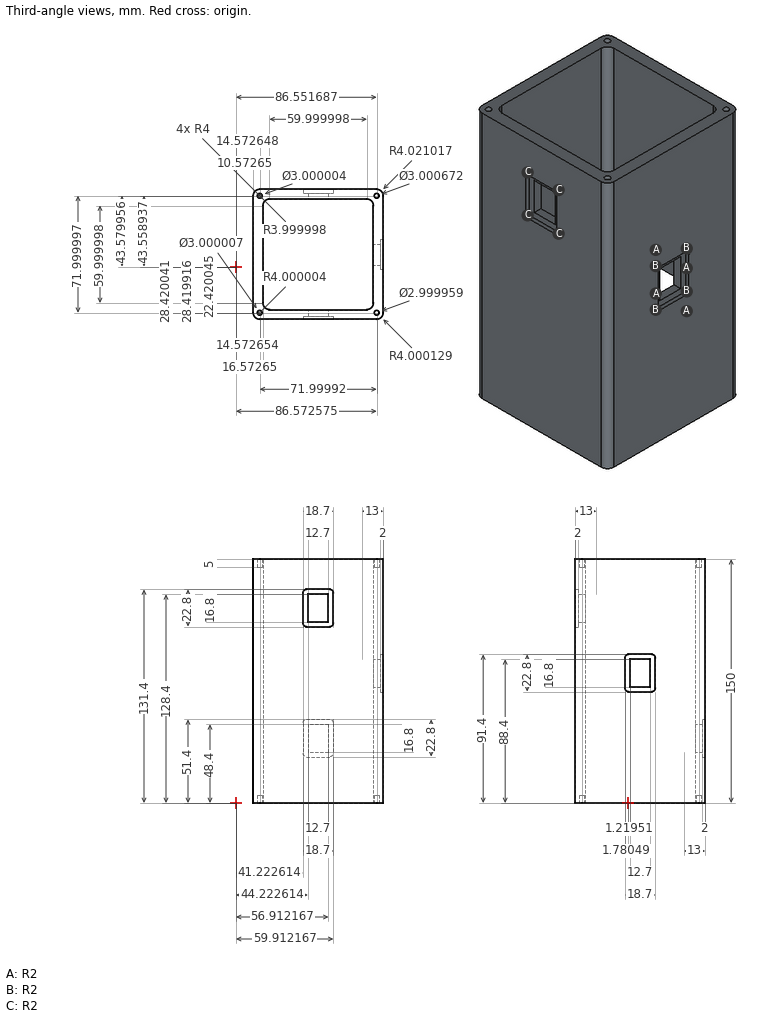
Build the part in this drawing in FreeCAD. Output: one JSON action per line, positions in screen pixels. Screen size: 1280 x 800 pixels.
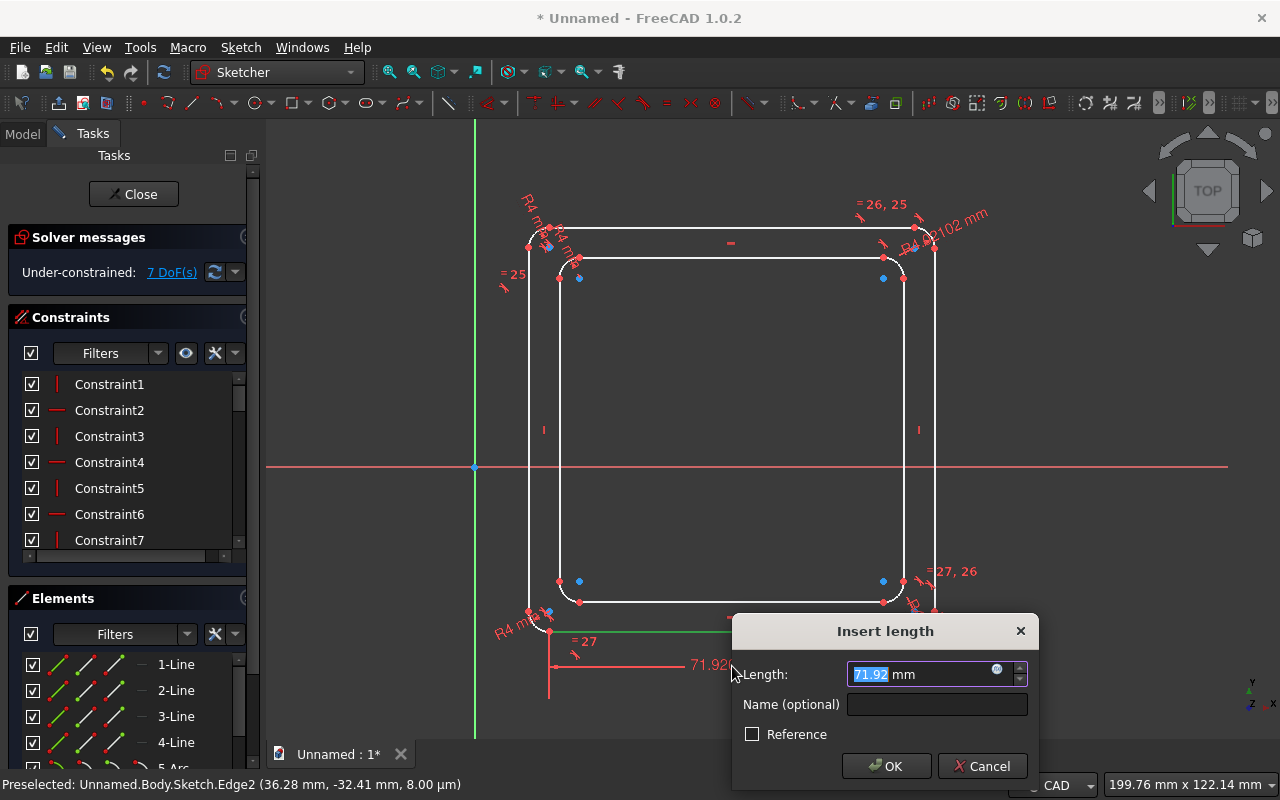
{"action": "type", "text": "71.99992"}
{"action": "key", "text": "Return"}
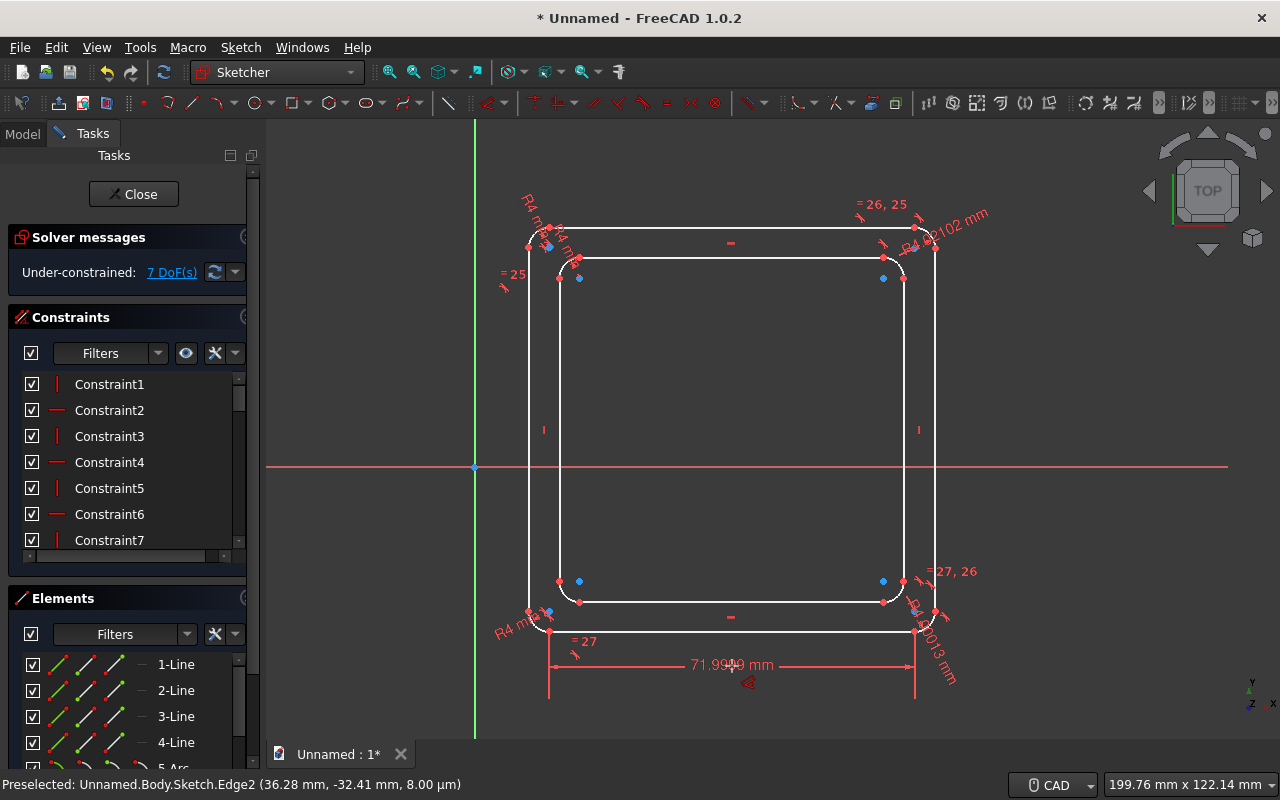
{"action": "left_click", "coordinate": [529, 357]}
{"action": "left_click", "coordinate": [495, 430]}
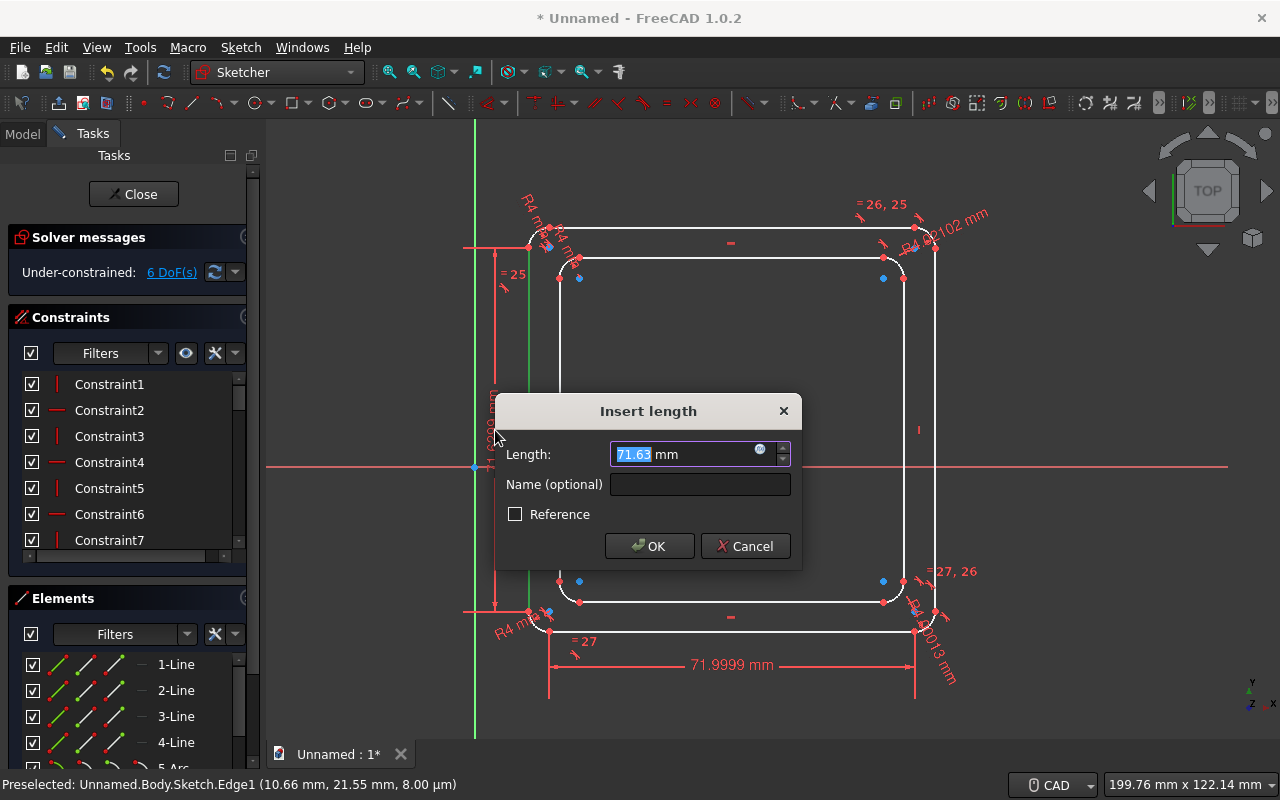
{"action": "type", "text": "71.999997"}
{"action": "key", "text": "Return"}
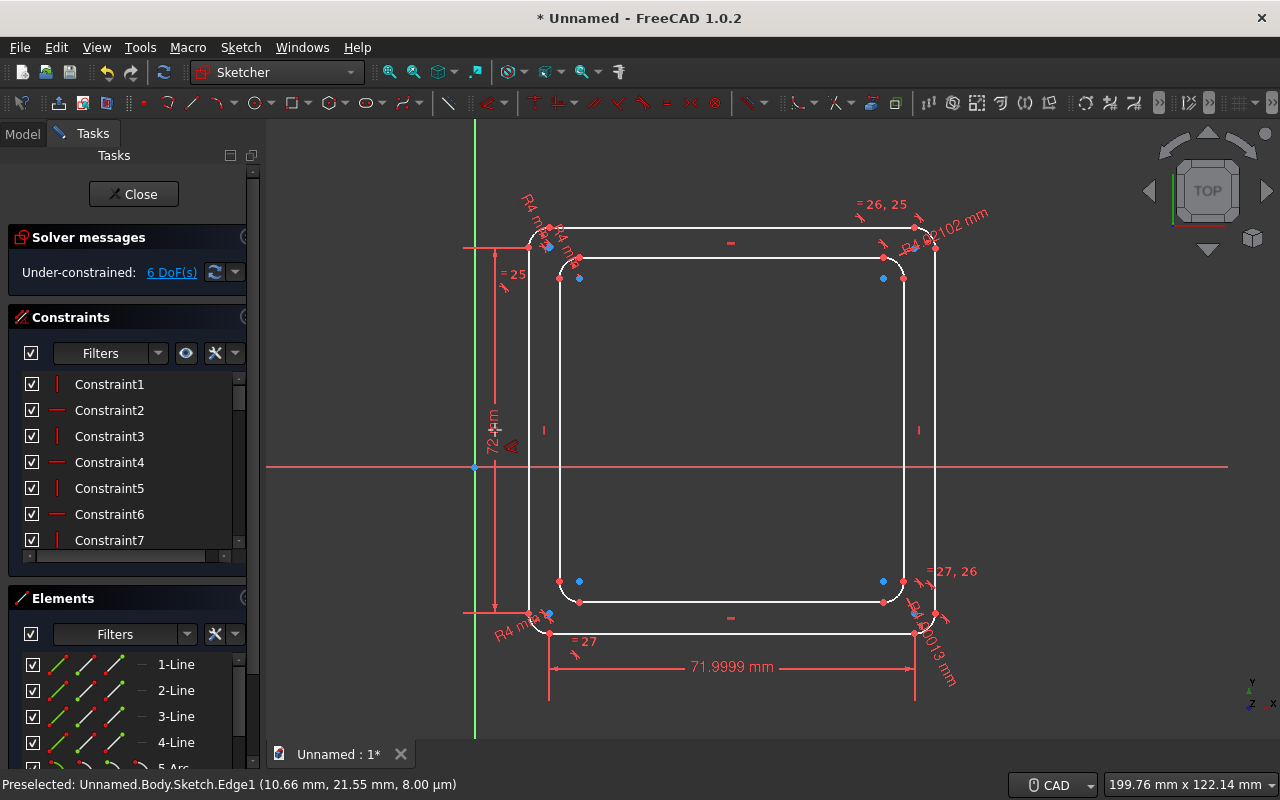
{"action": "left_click", "coordinate": [560, 491]}
{"action": "left_click", "coordinate": [594, 430]}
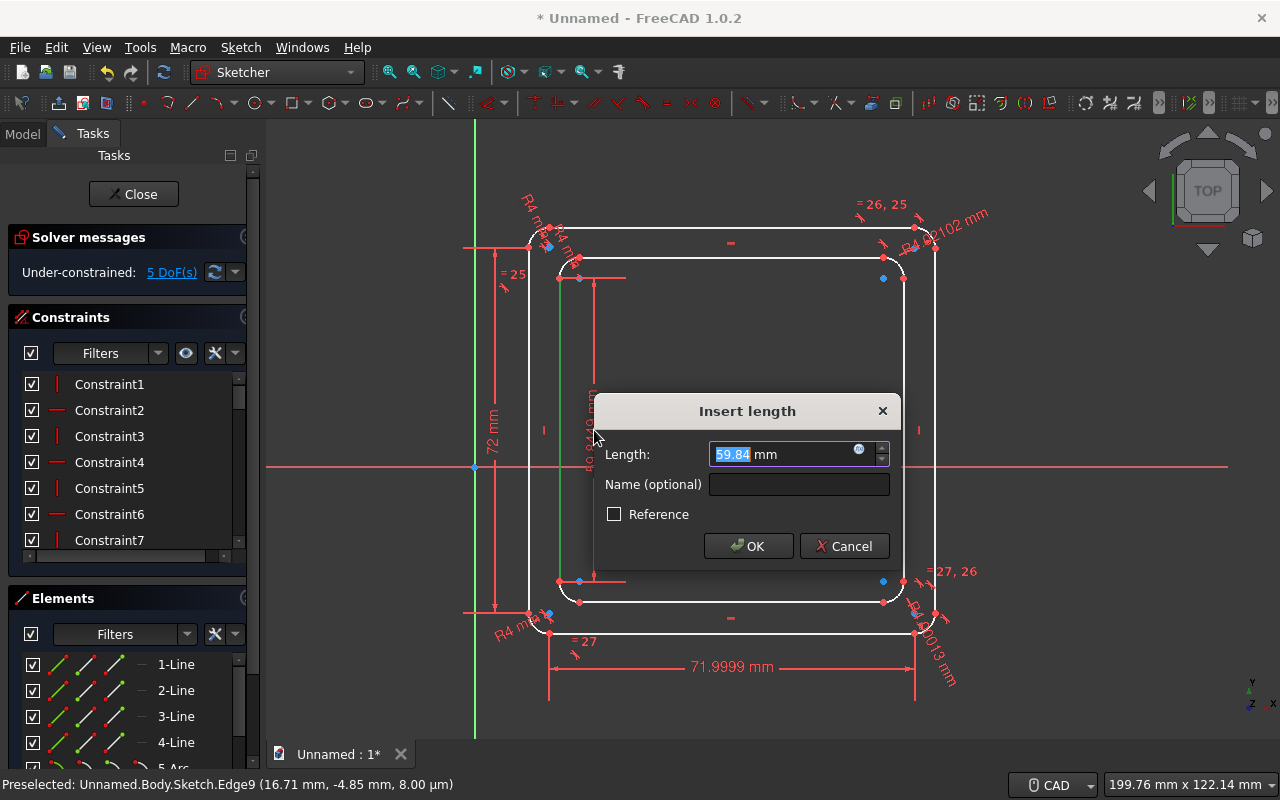
{"action": "type", "text": "59.999998"}
{"action": "key", "text": "Return"}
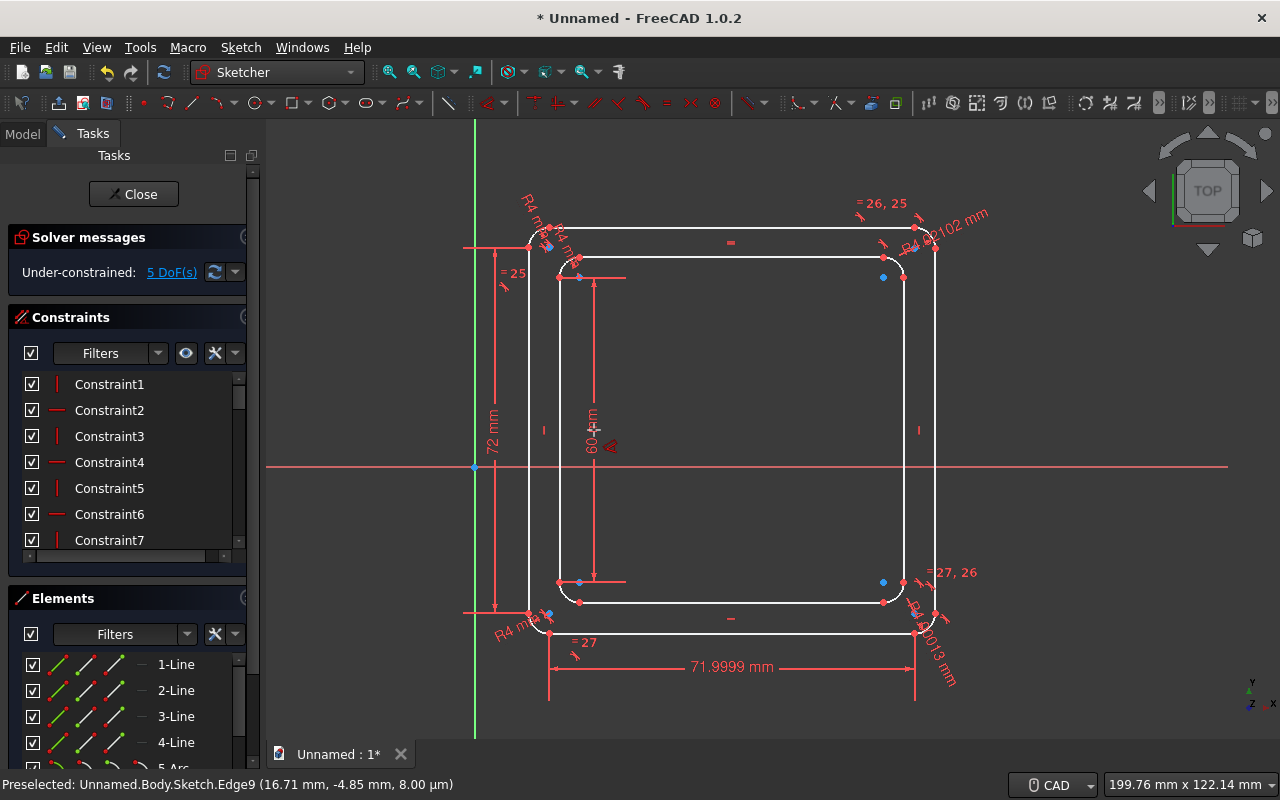
{"action": "left_click", "coordinate": [671, 257]}
{"action": "left_click", "coordinate": [732, 291]}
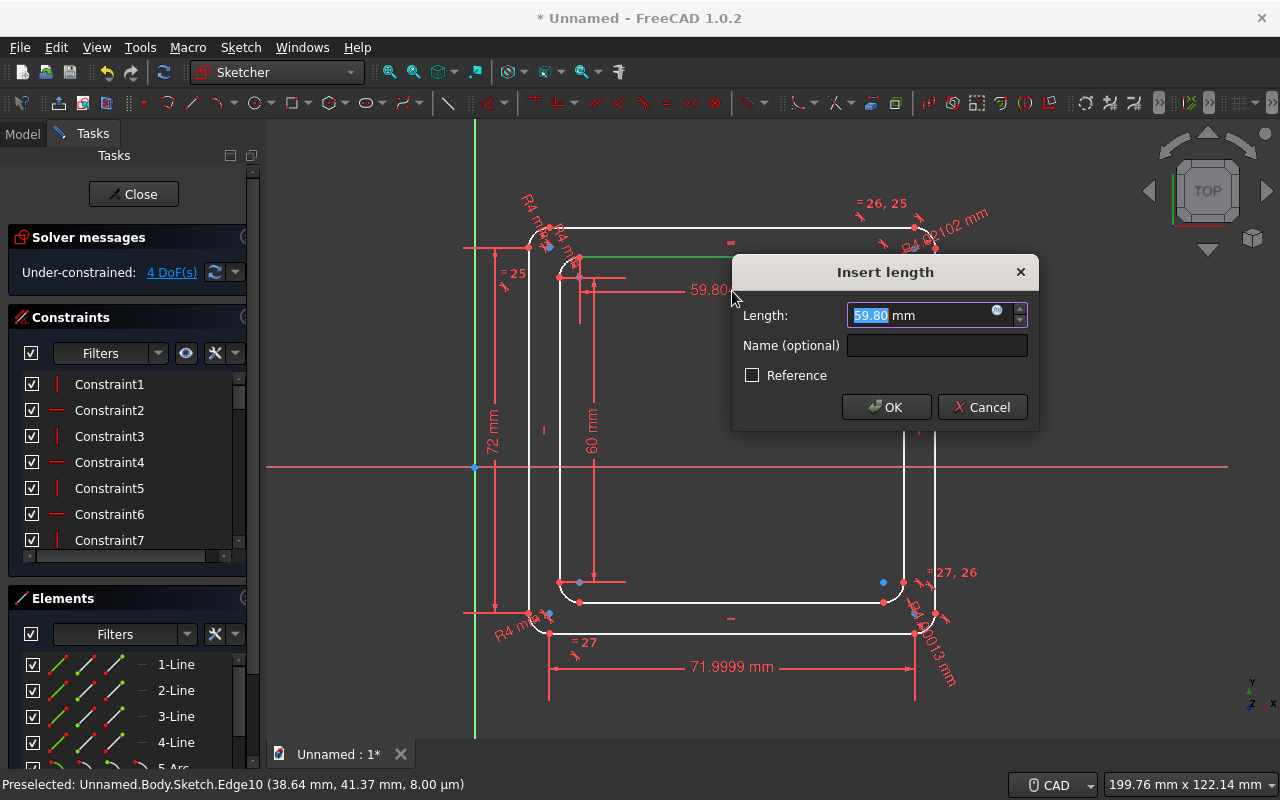
{"action": "type", "text": "59.999998"}
{"action": "key", "text": "Return"}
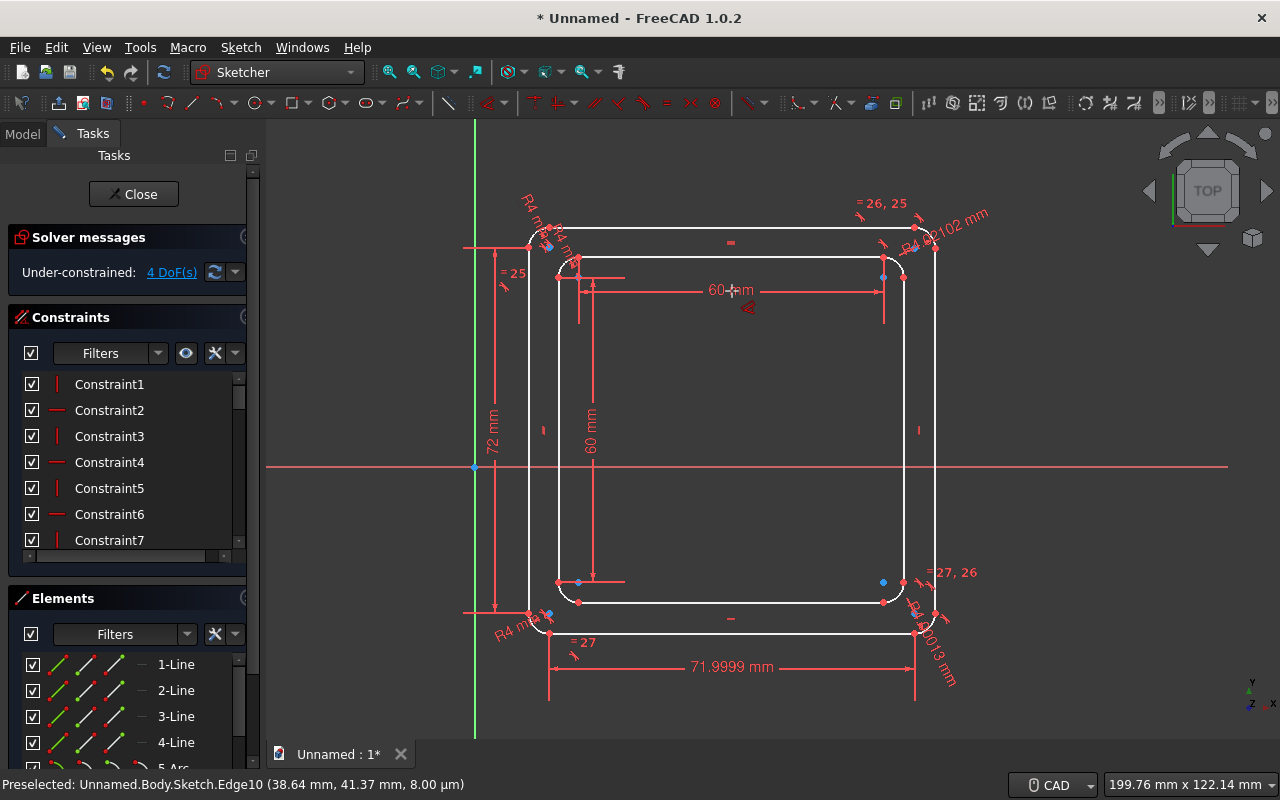
{"action": "left_click", "coordinate": [529, 248]}
{"action": "left_click", "coordinate": [502, 501]}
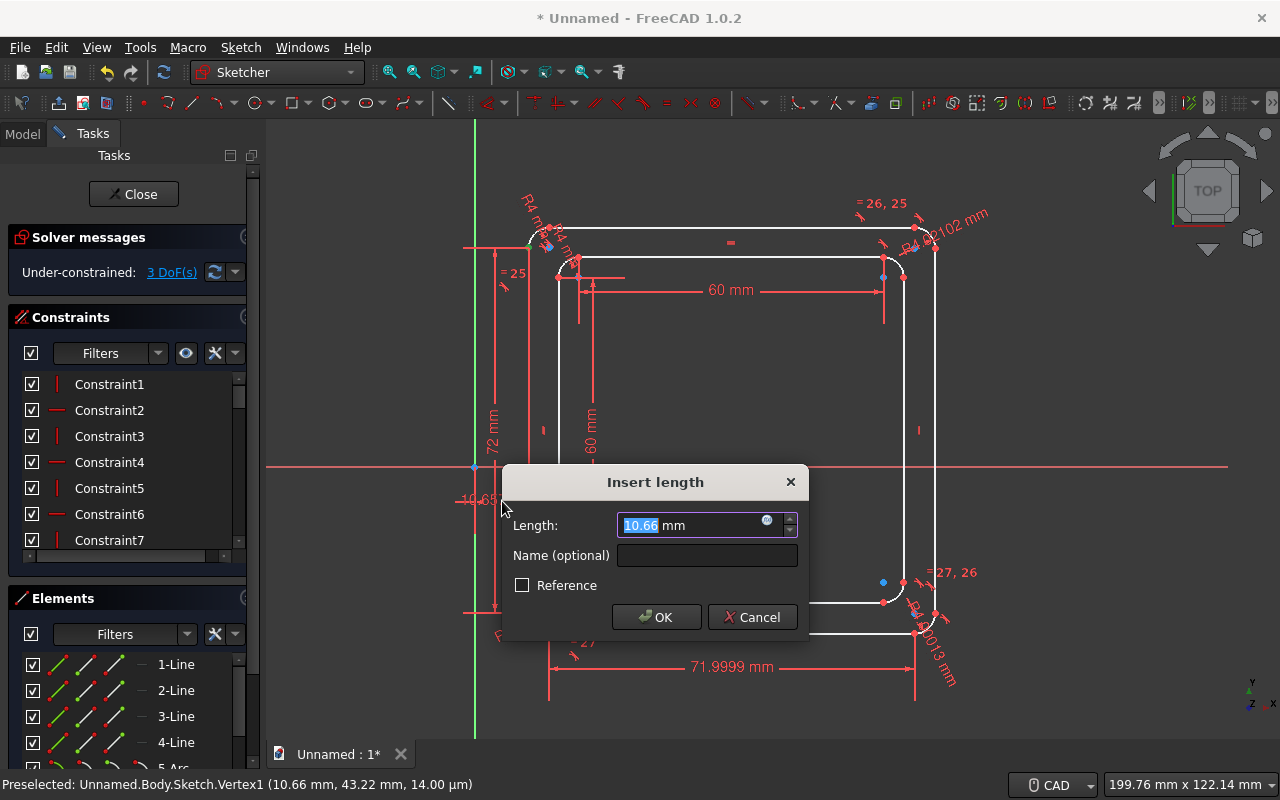
{"action": "type", "text": "10.57265"}
{"action": "key", "text": "Return"}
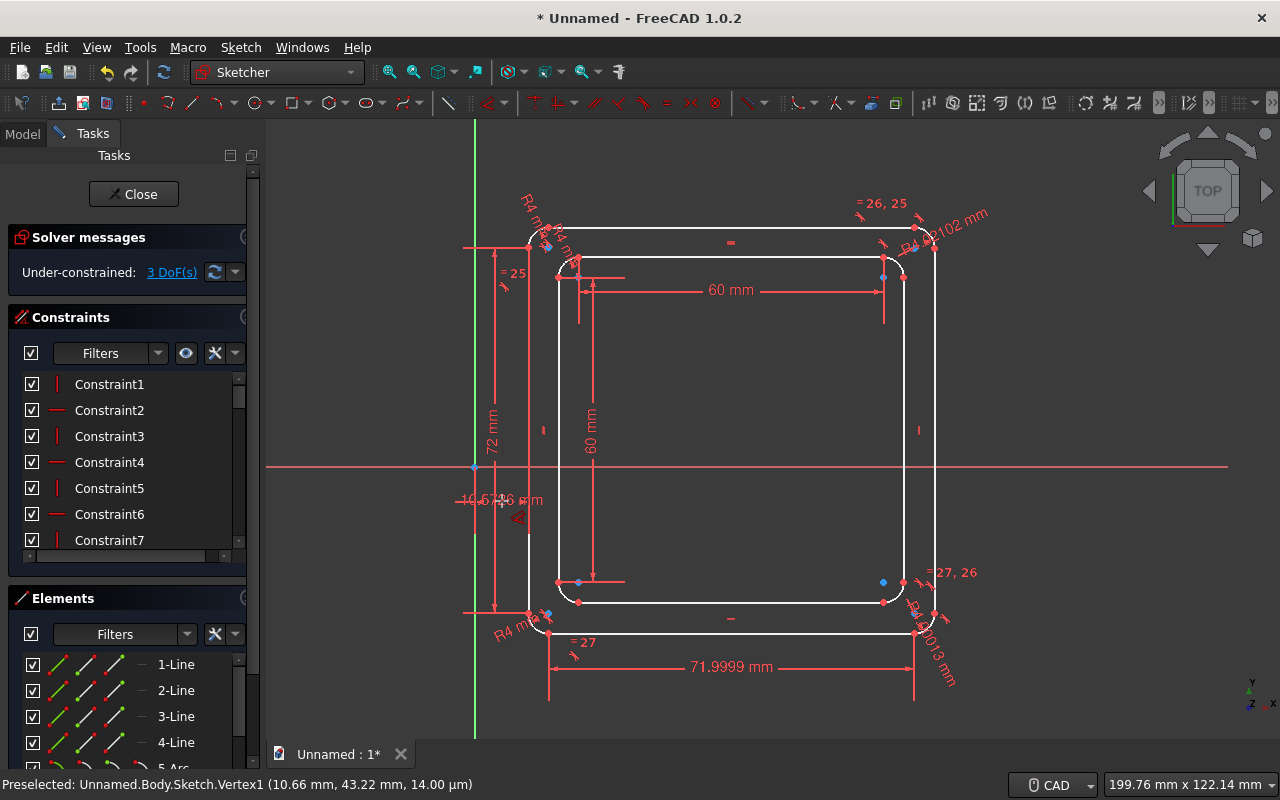
{"action": "left_click", "coordinate": [559, 582]}
{"action": "left_click", "coordinate": [497, 409]}